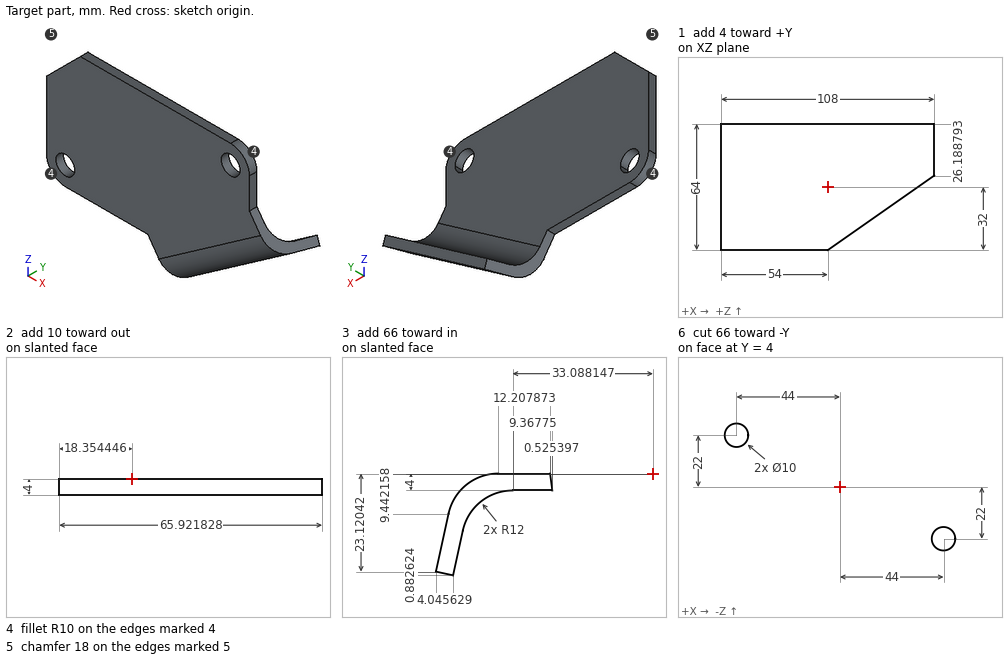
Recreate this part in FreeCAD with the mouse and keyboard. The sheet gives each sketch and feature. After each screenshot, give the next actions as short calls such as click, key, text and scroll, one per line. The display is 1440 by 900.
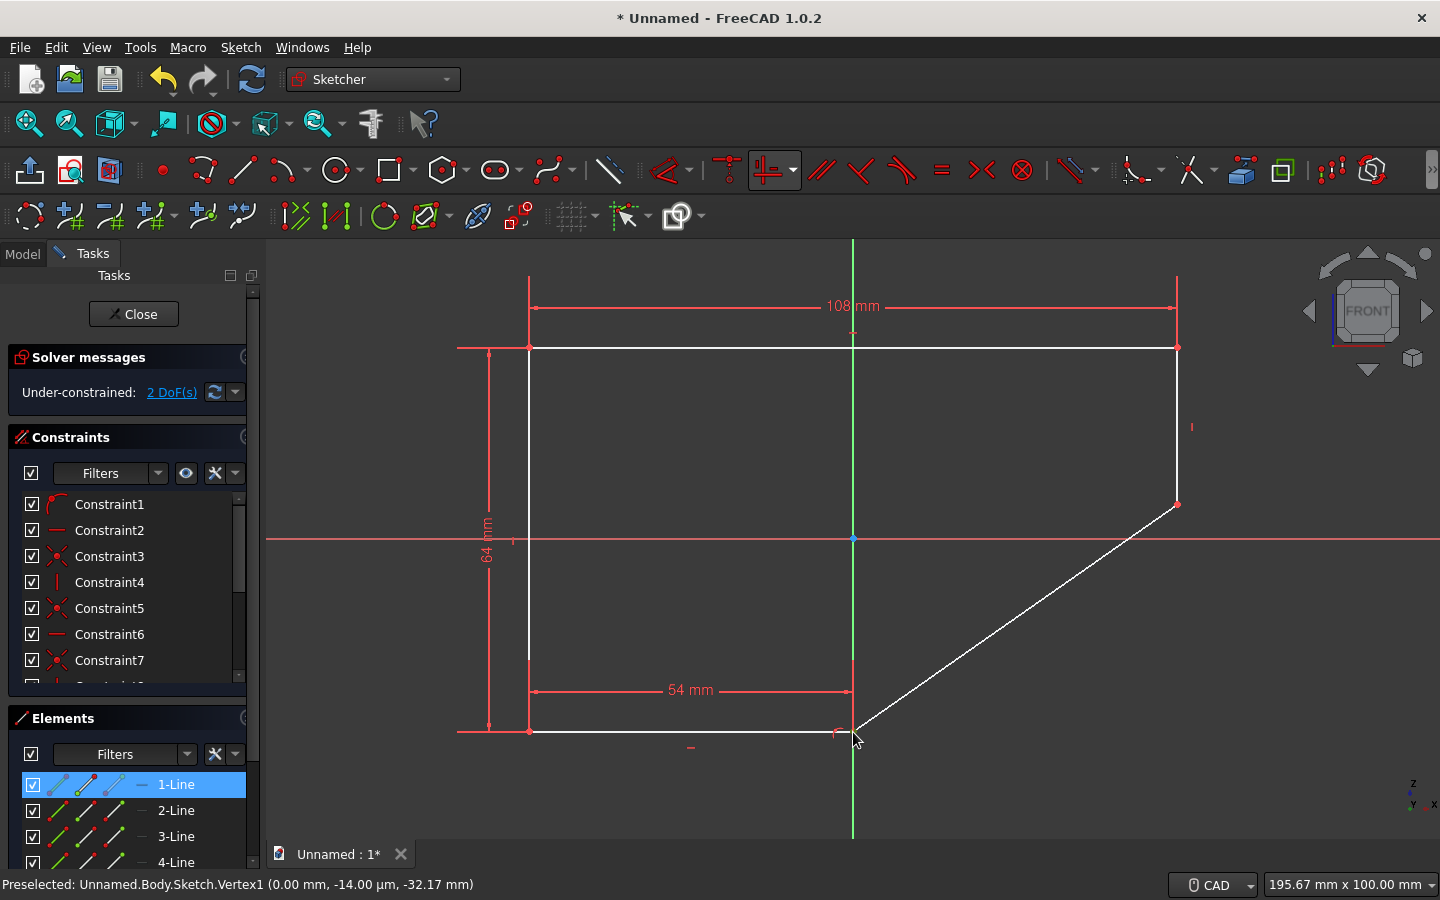
key(i)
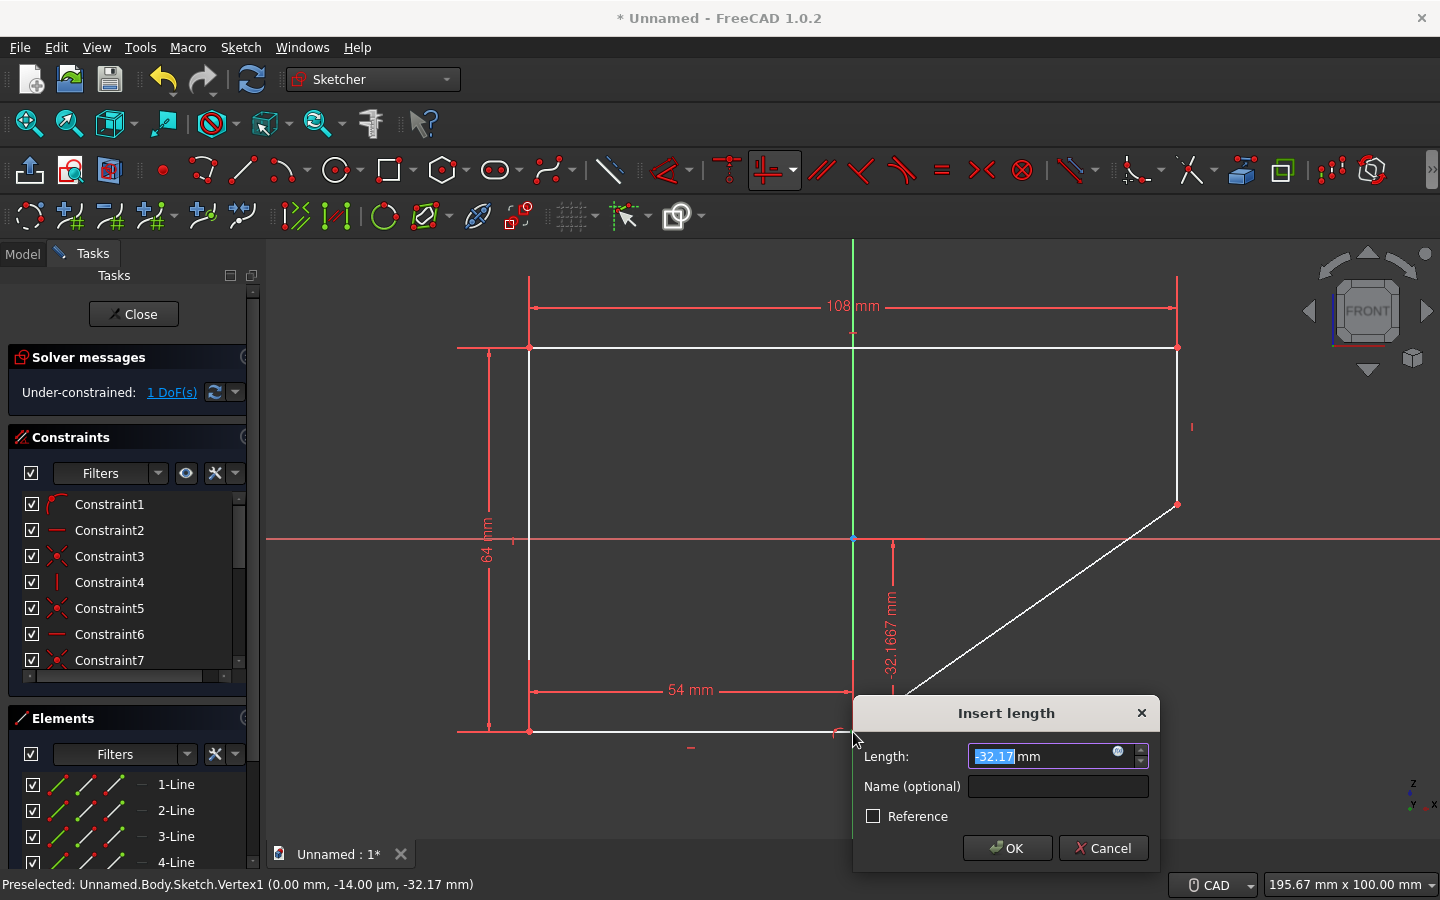
text(-32)
key(Return)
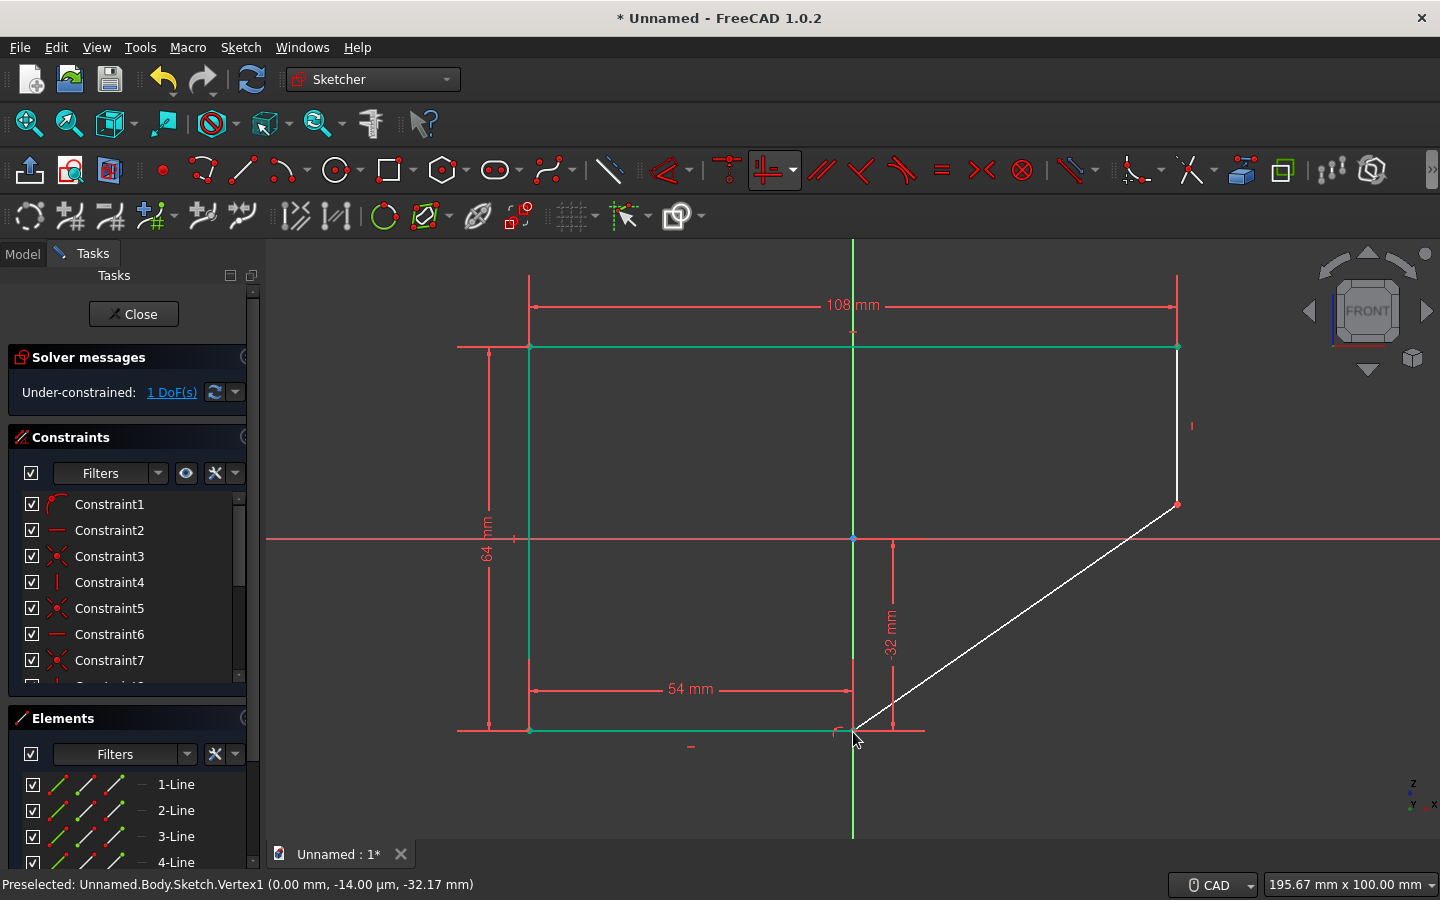
click(1177, 394)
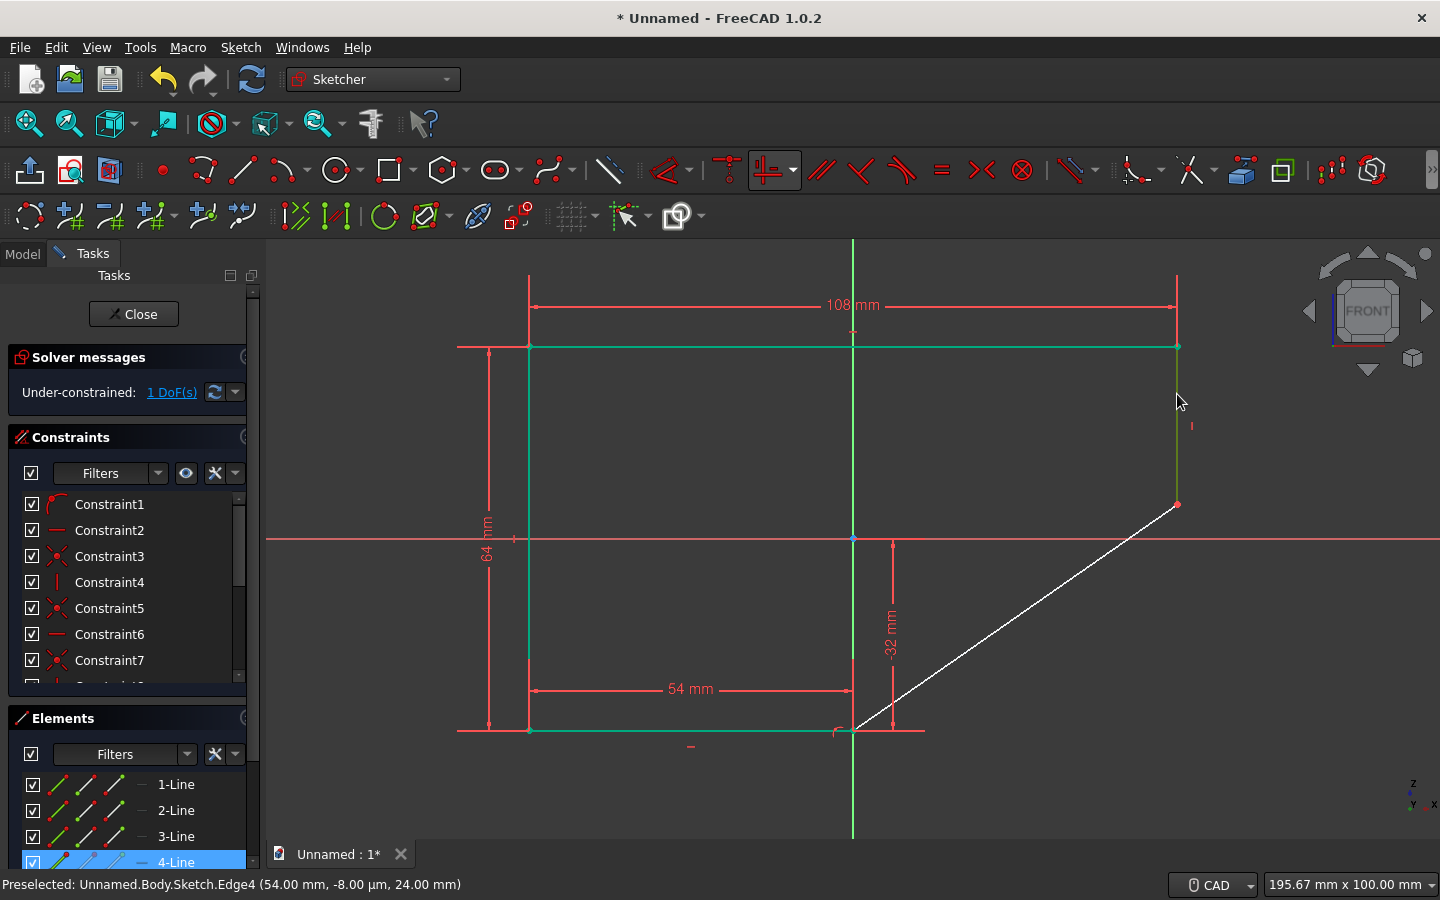
key(i)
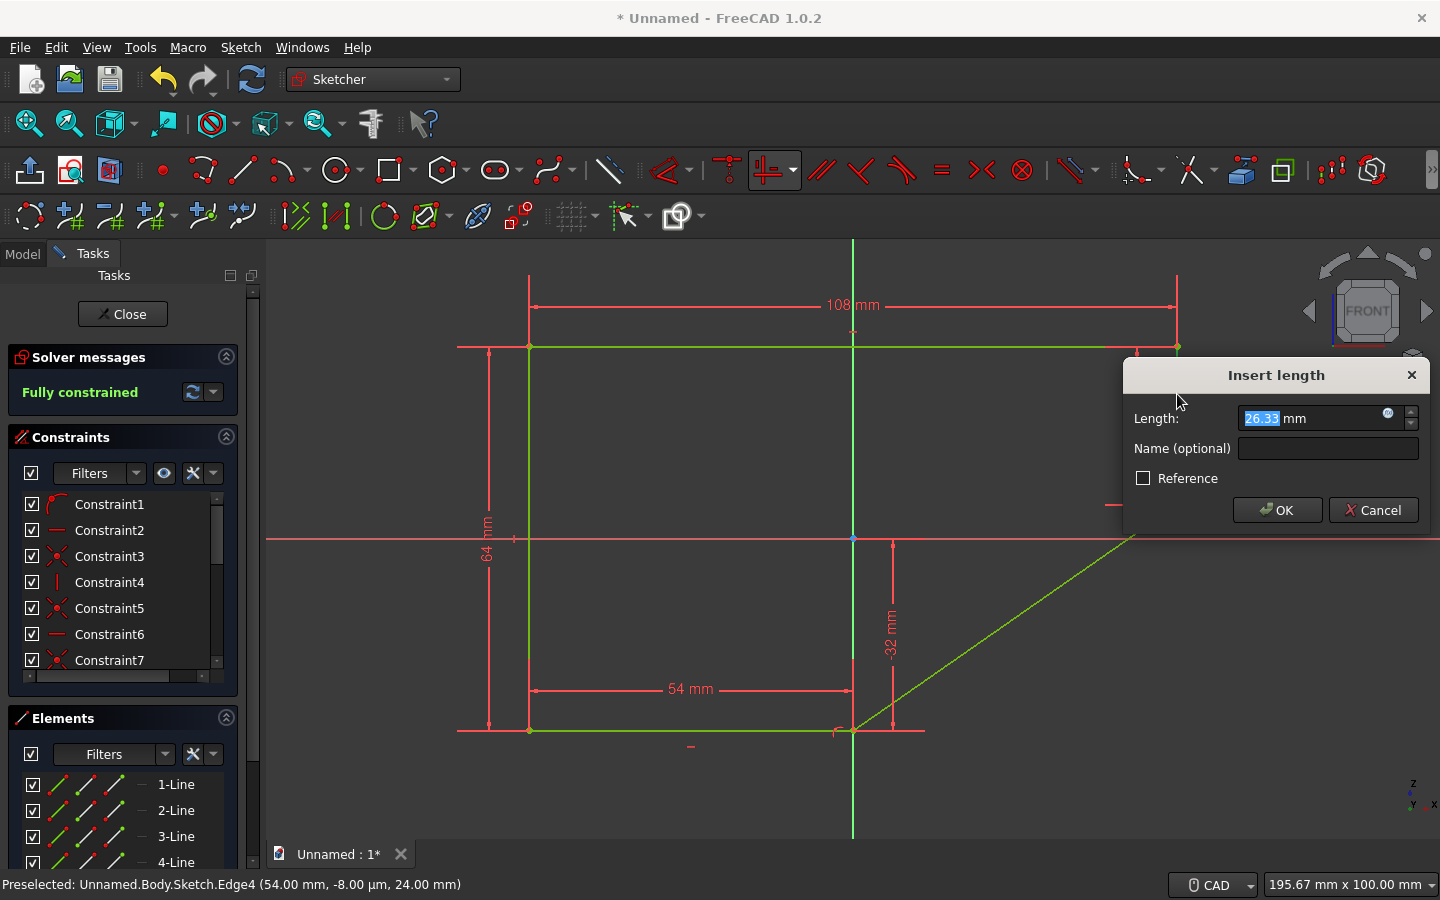
text(26.188793)
key(Return)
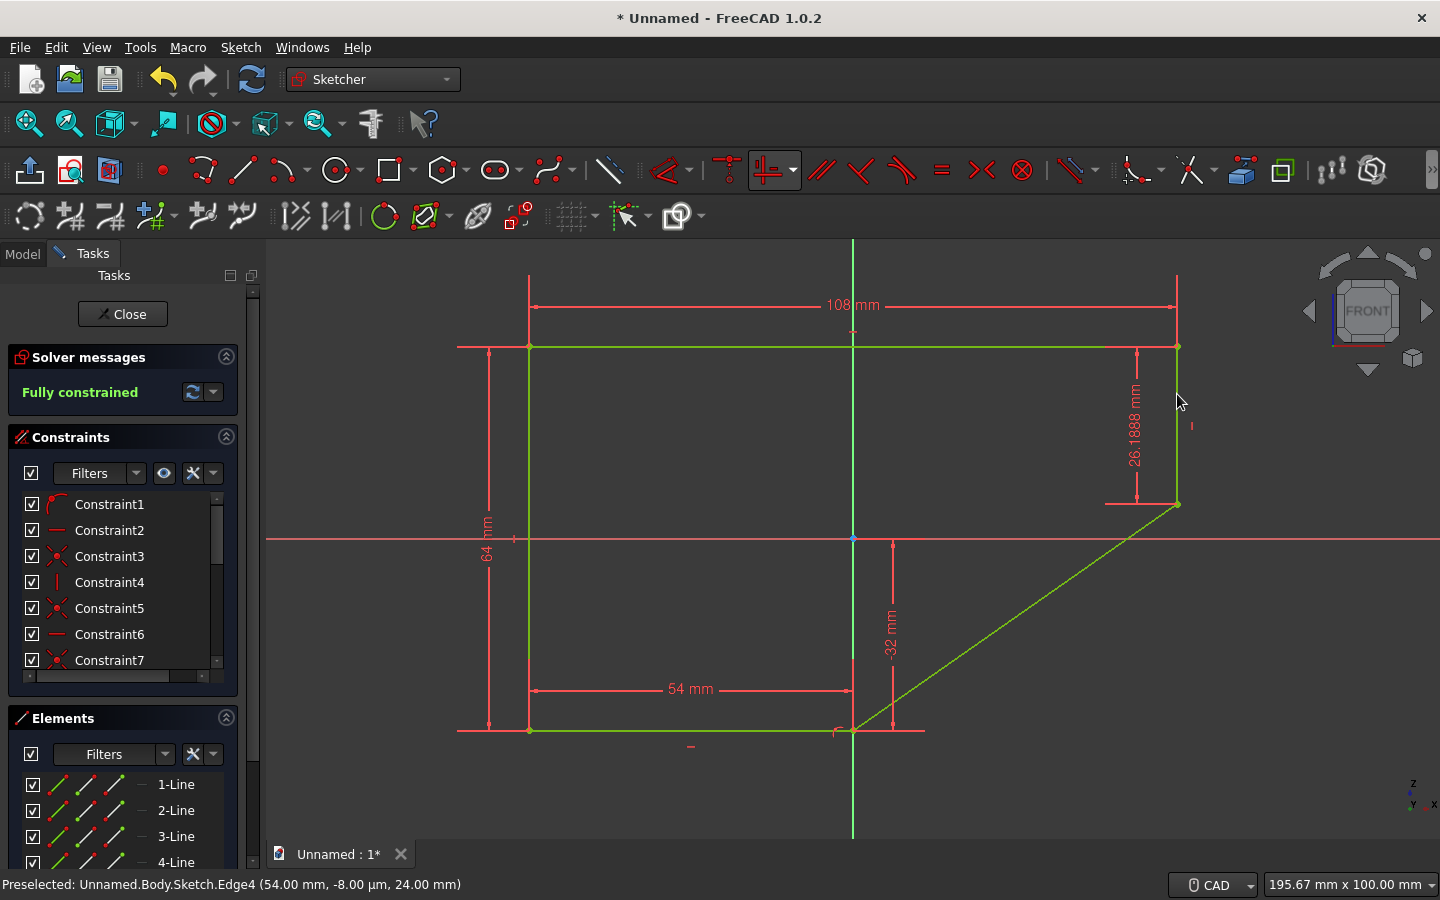
click(123, 314)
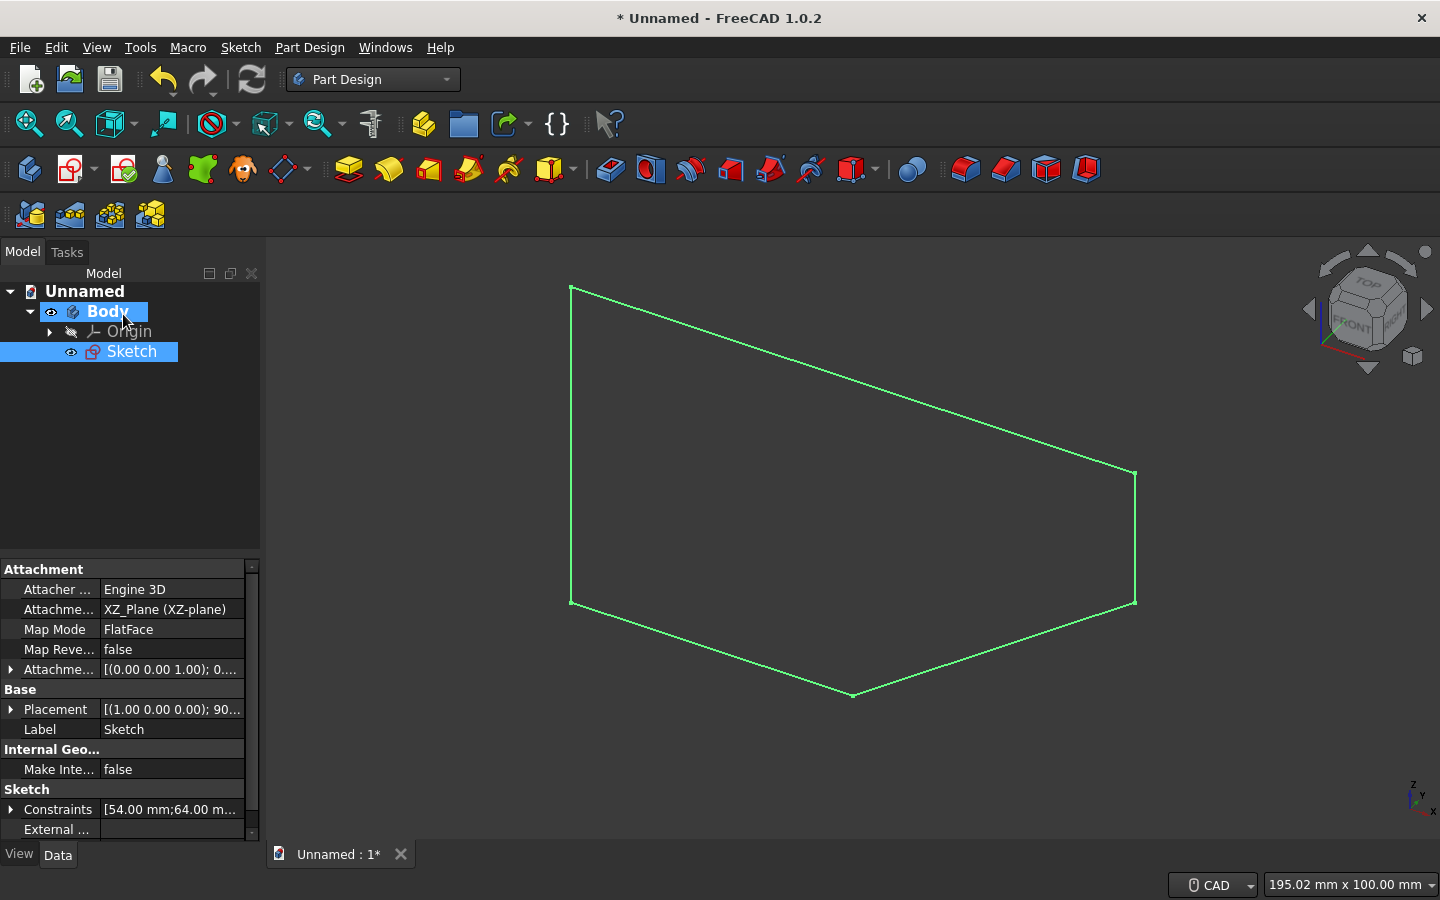
click(350, 170)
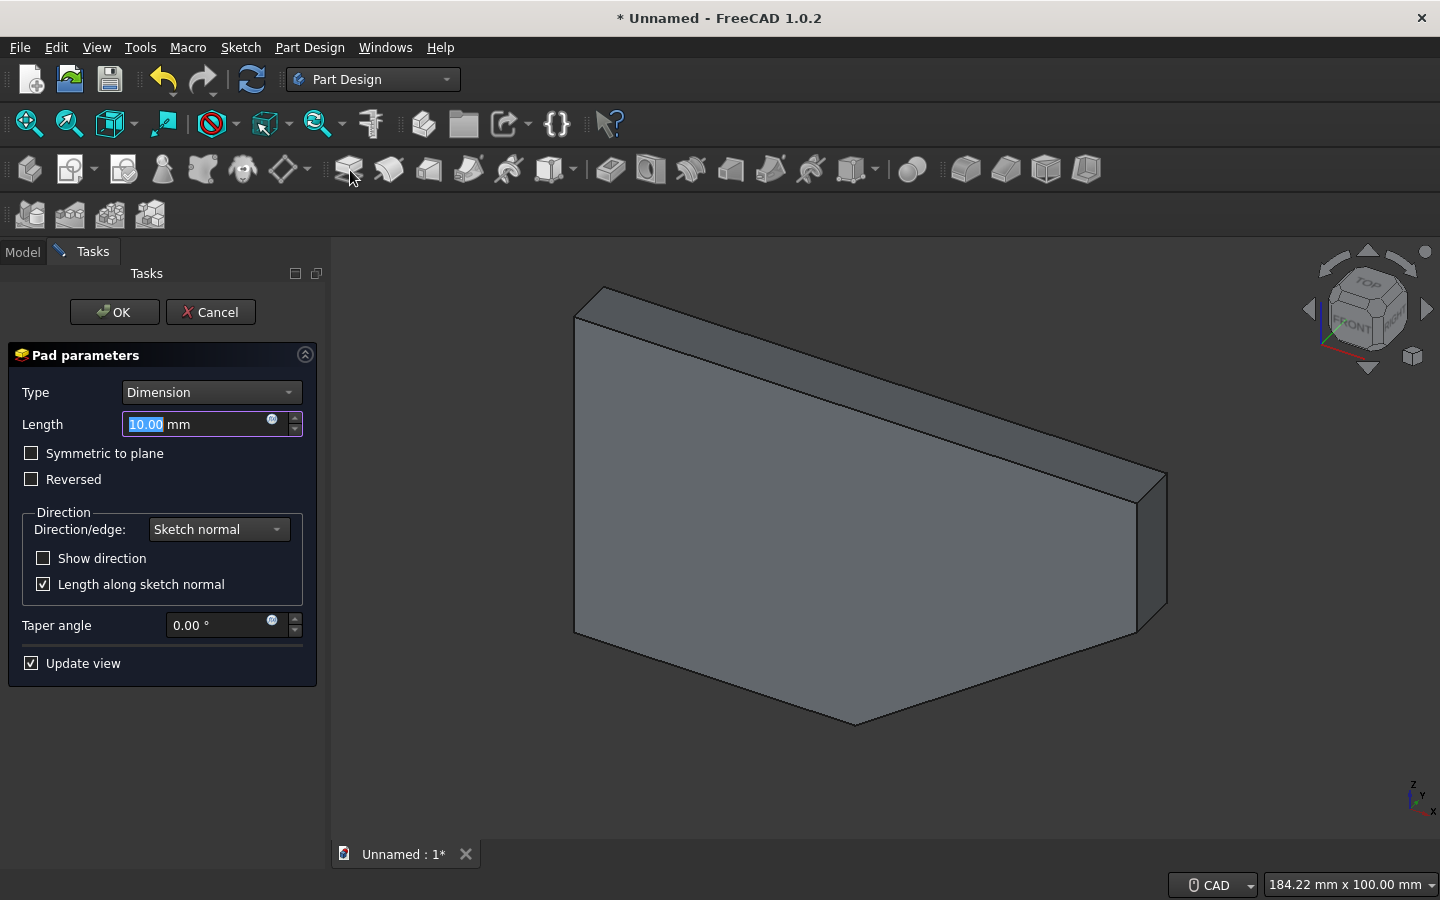
text(4)
key(Tab)